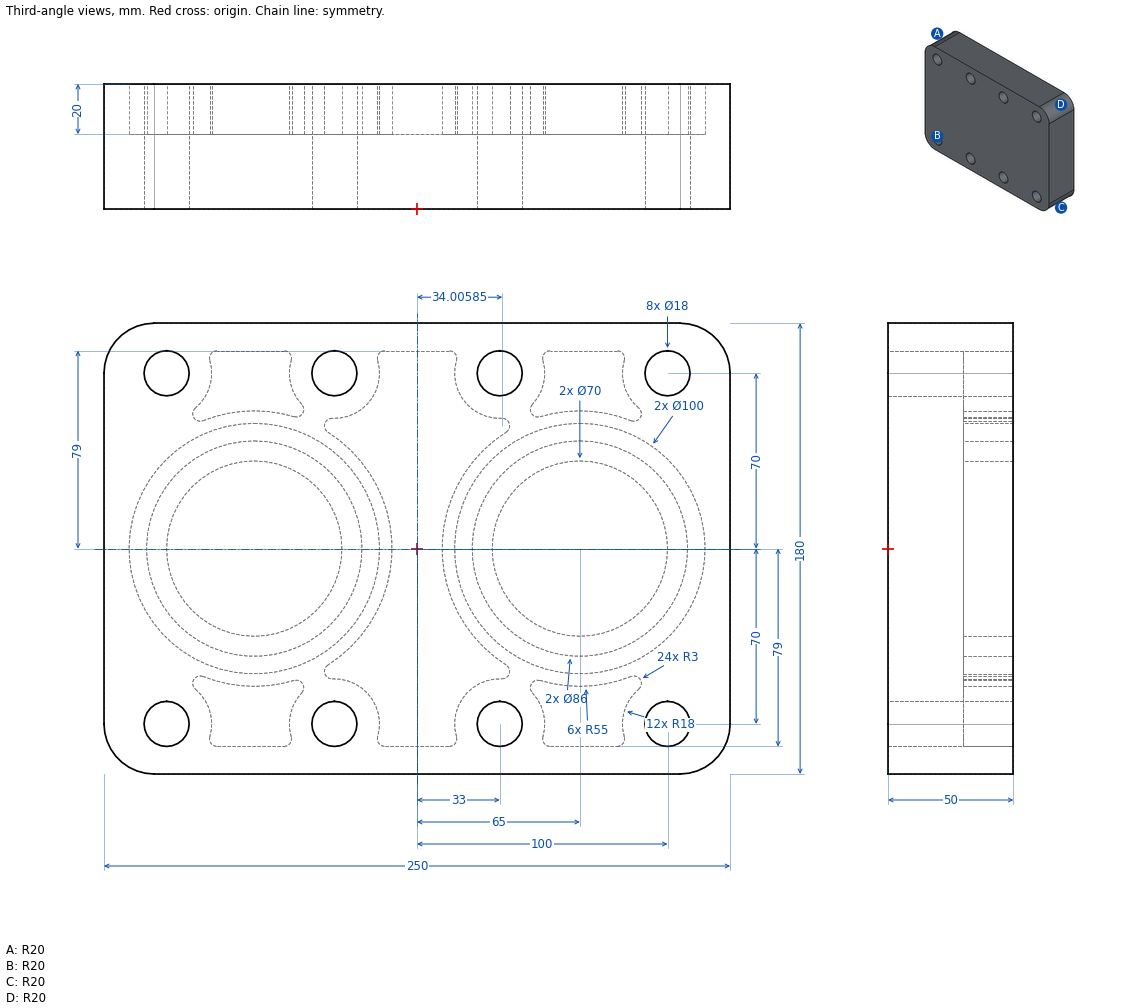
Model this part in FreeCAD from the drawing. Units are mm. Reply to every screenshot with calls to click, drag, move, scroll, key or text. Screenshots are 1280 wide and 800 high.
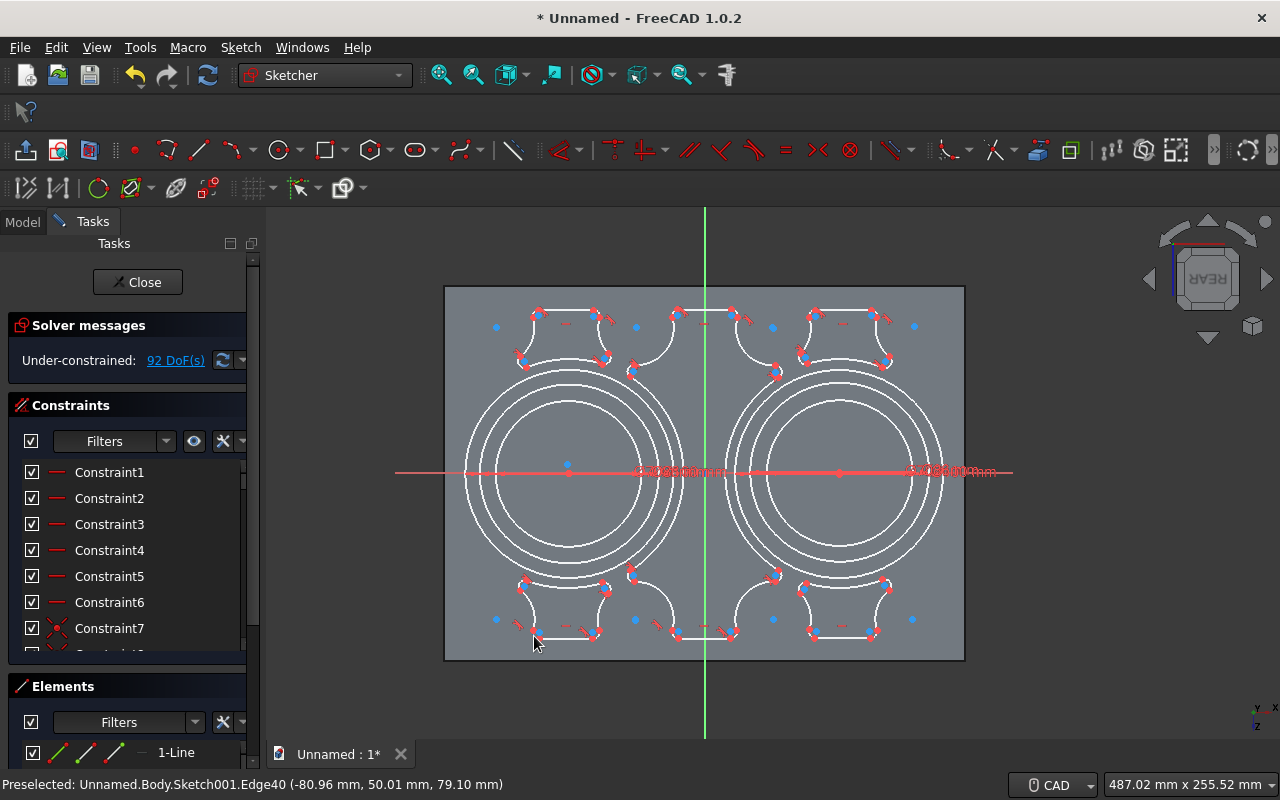
click(832, 638)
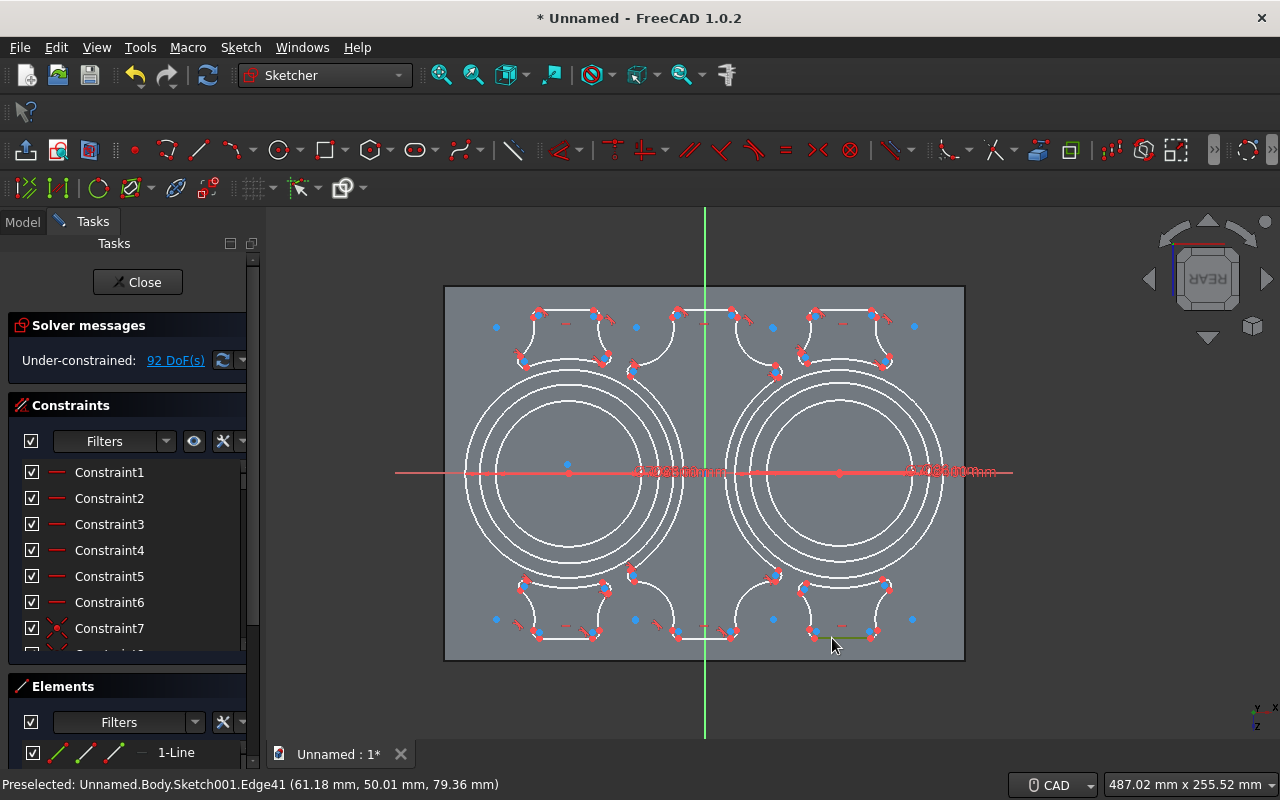
scroll(876, 636, up, 5)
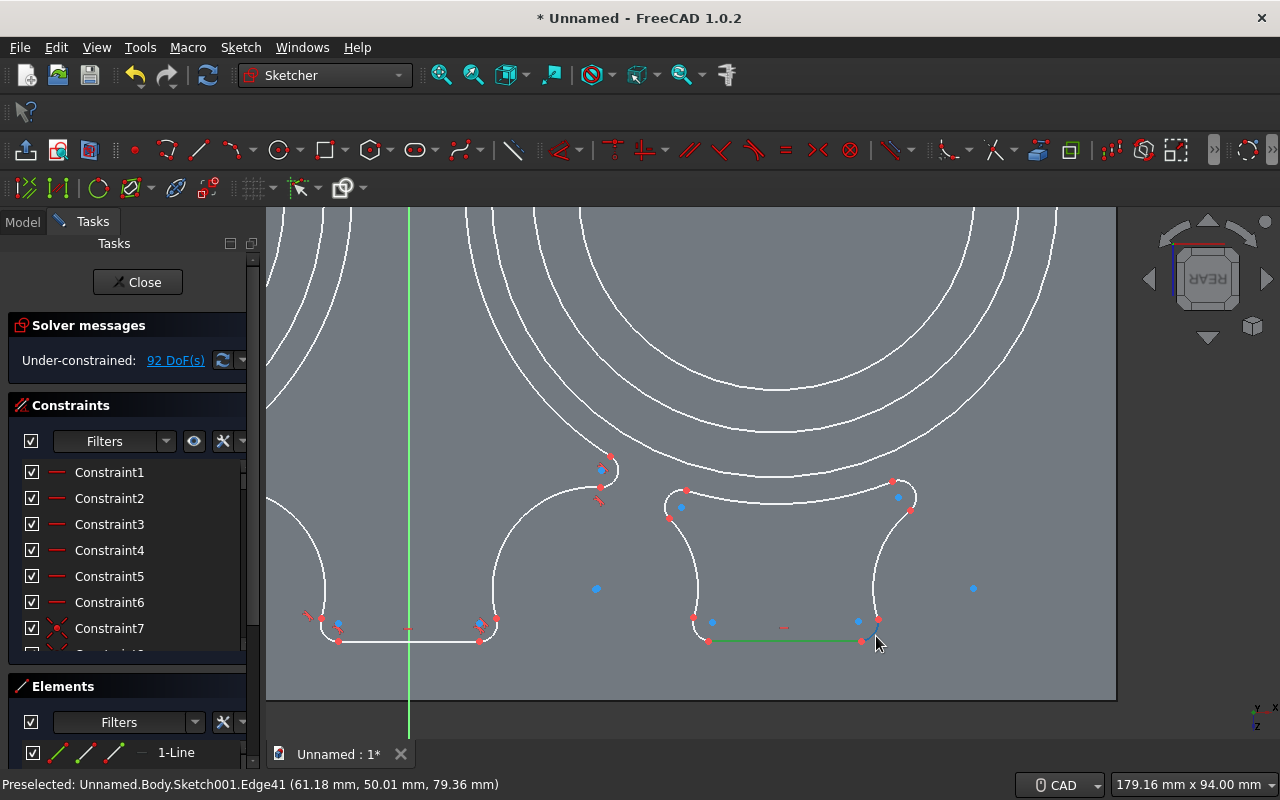
click(874, 634)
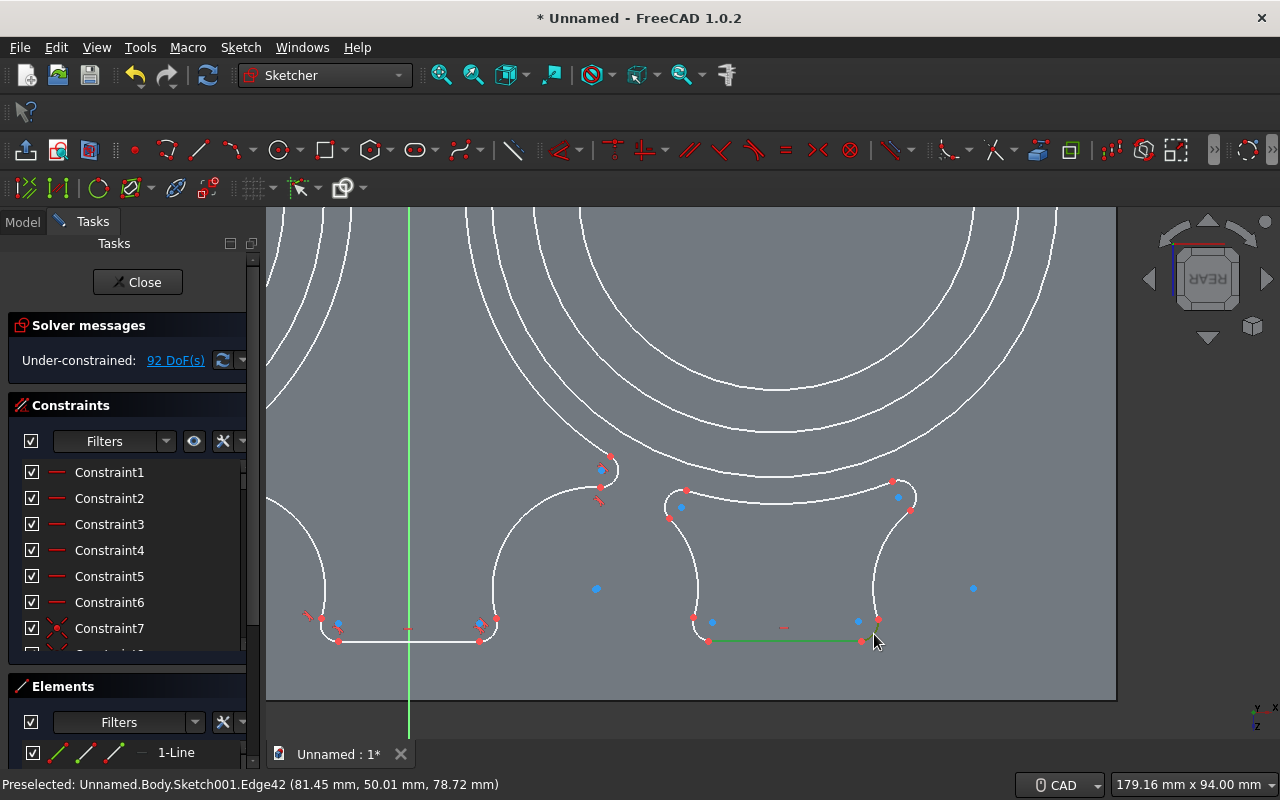
click(754, 150)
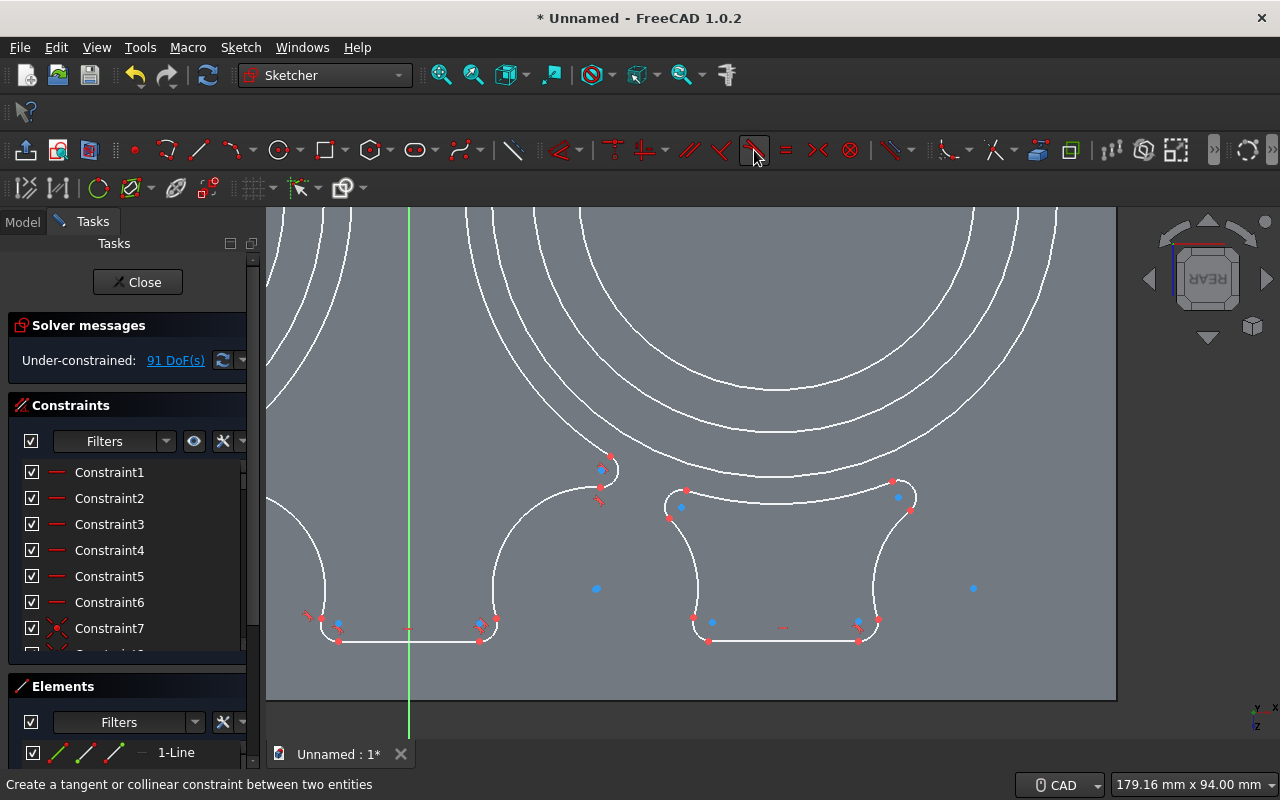
click(754, 641)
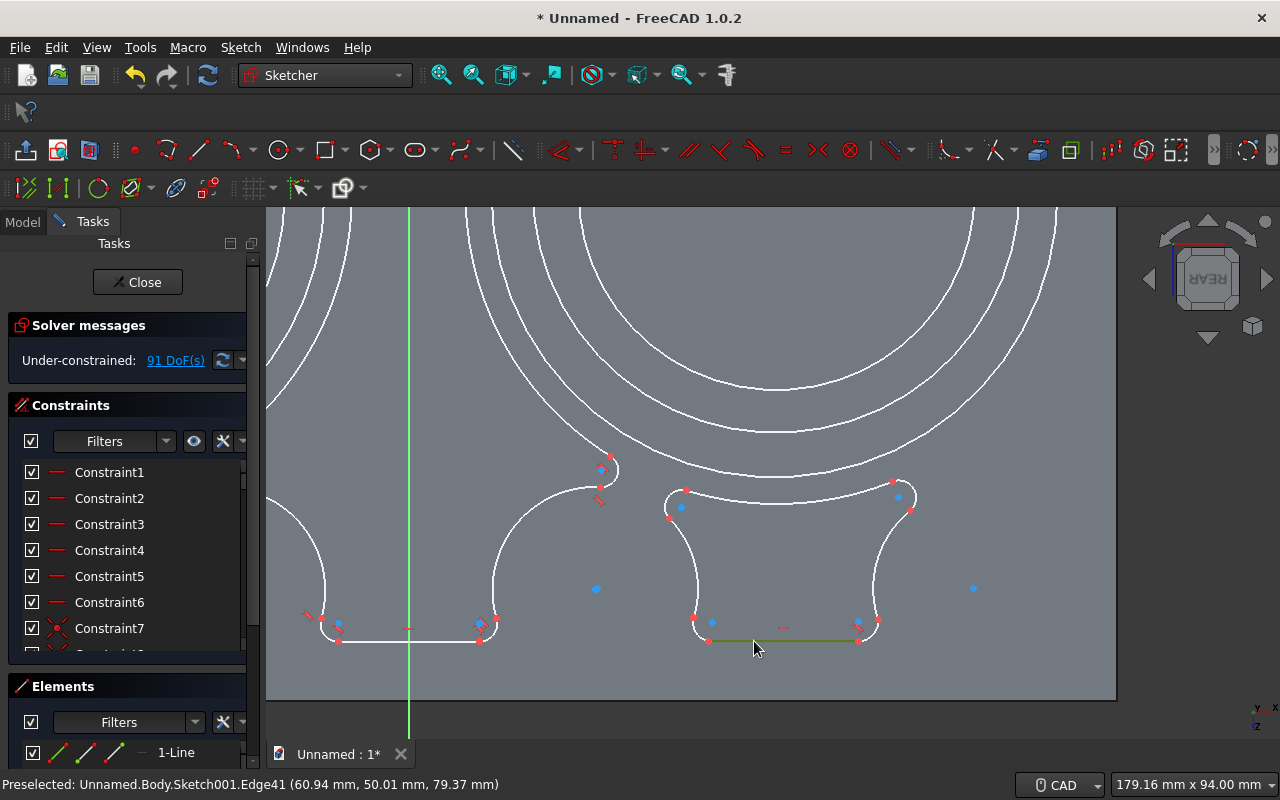
scroll(694, 627, up, 2)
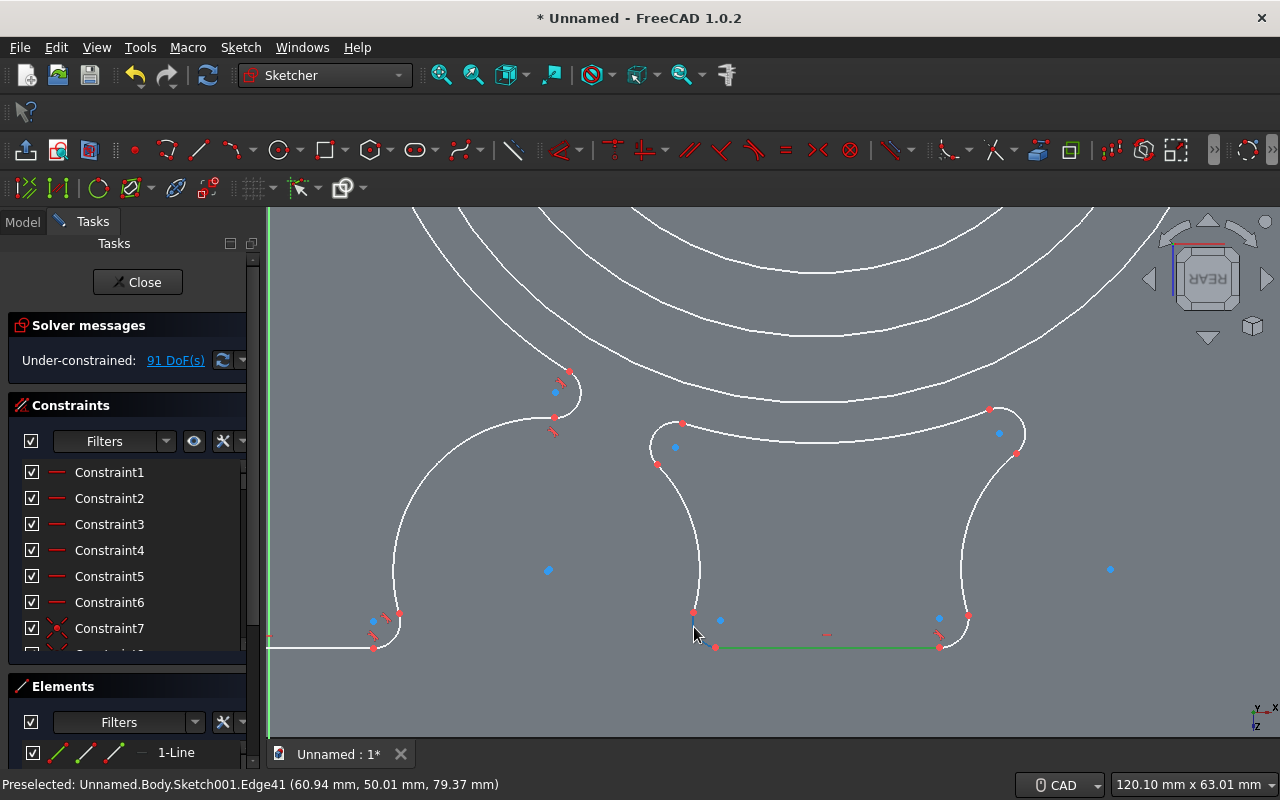
click(693, 627)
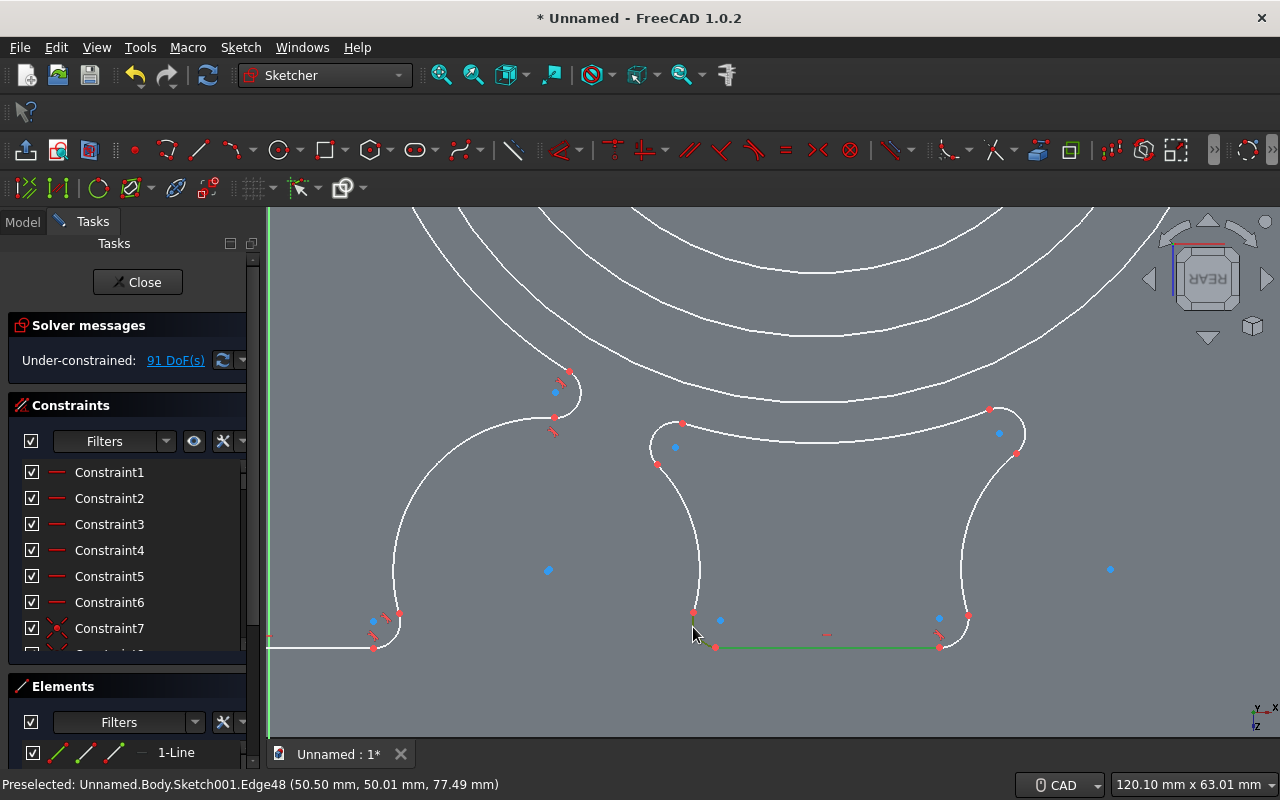
click(754, 150)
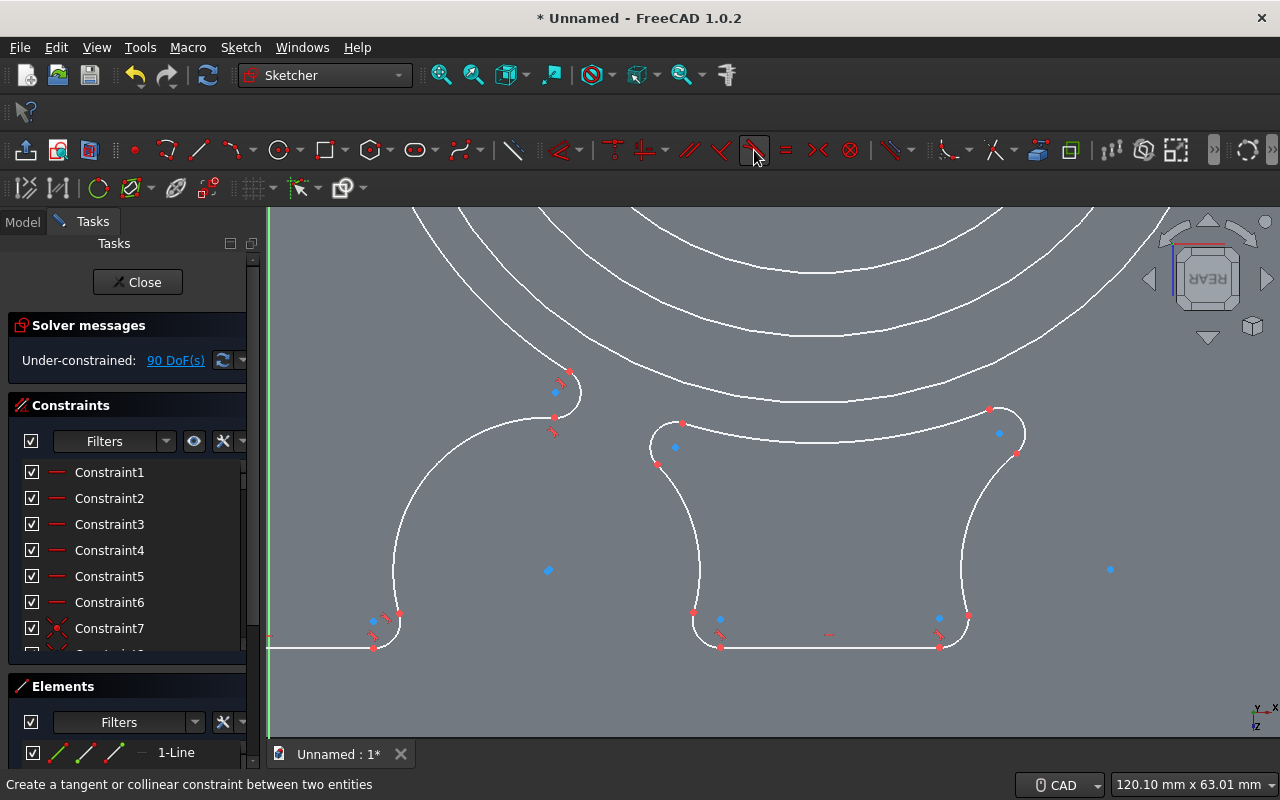
click(953, 644)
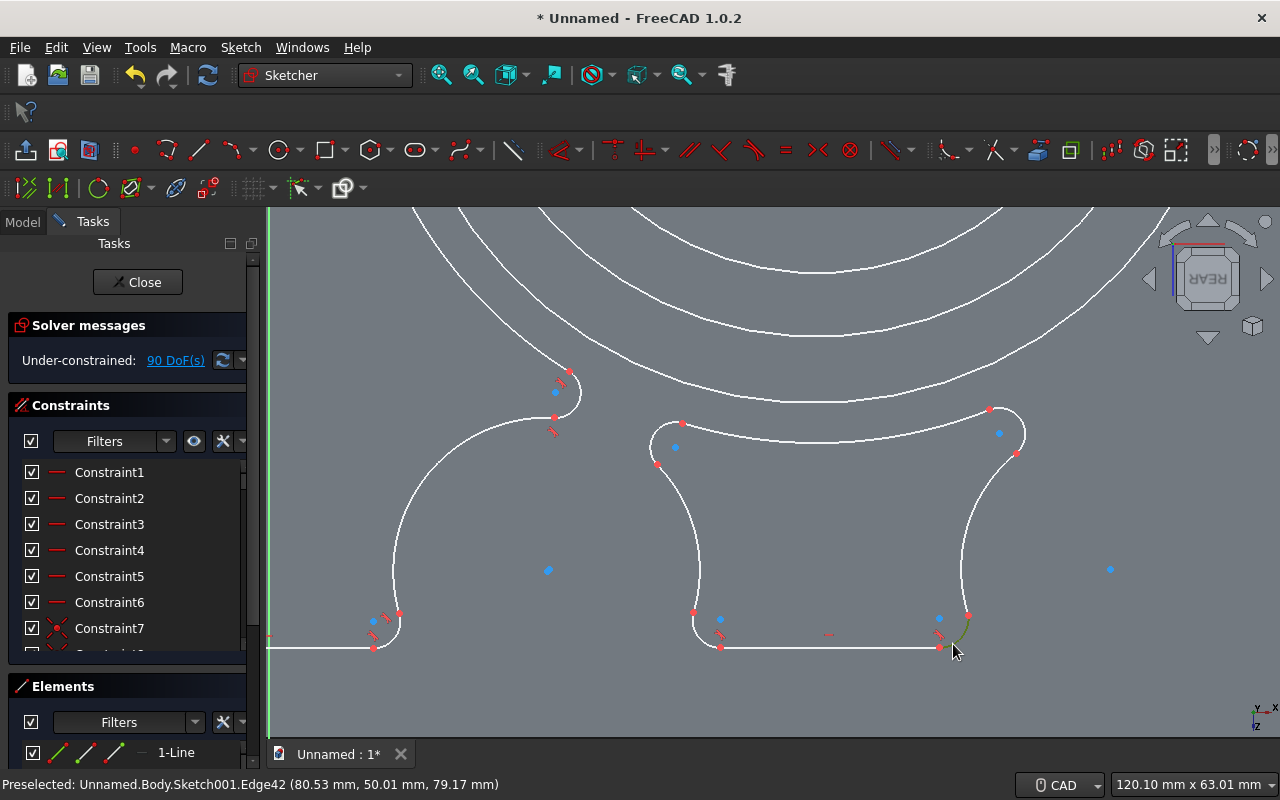
scroll(847, 635, down, 7)